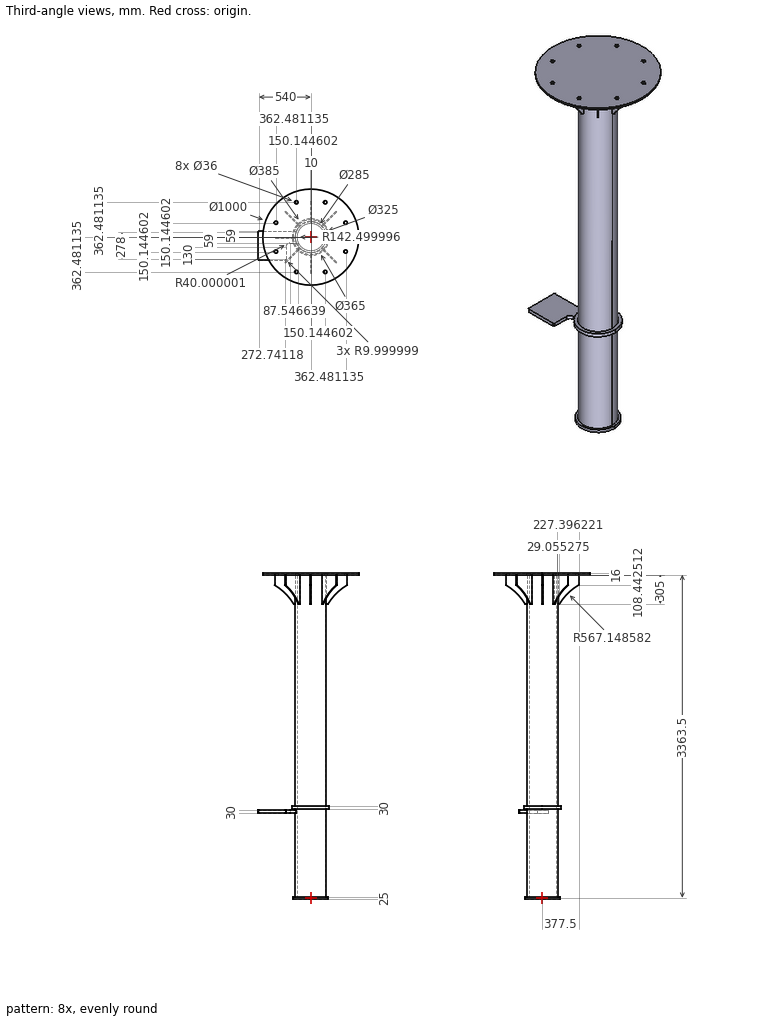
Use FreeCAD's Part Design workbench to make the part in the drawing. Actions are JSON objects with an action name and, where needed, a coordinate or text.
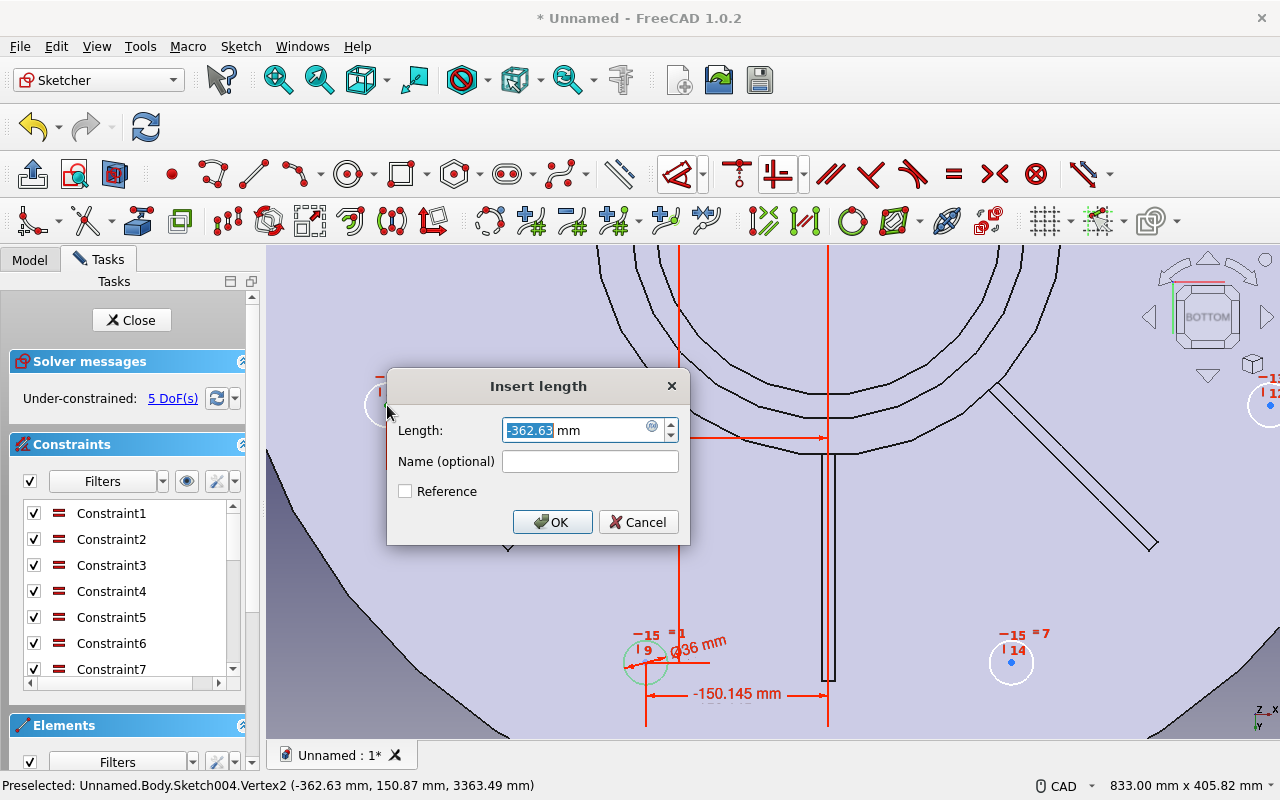
{"action": "type", "text": "-362.481135"}
{"action": "key", "text": "Return"}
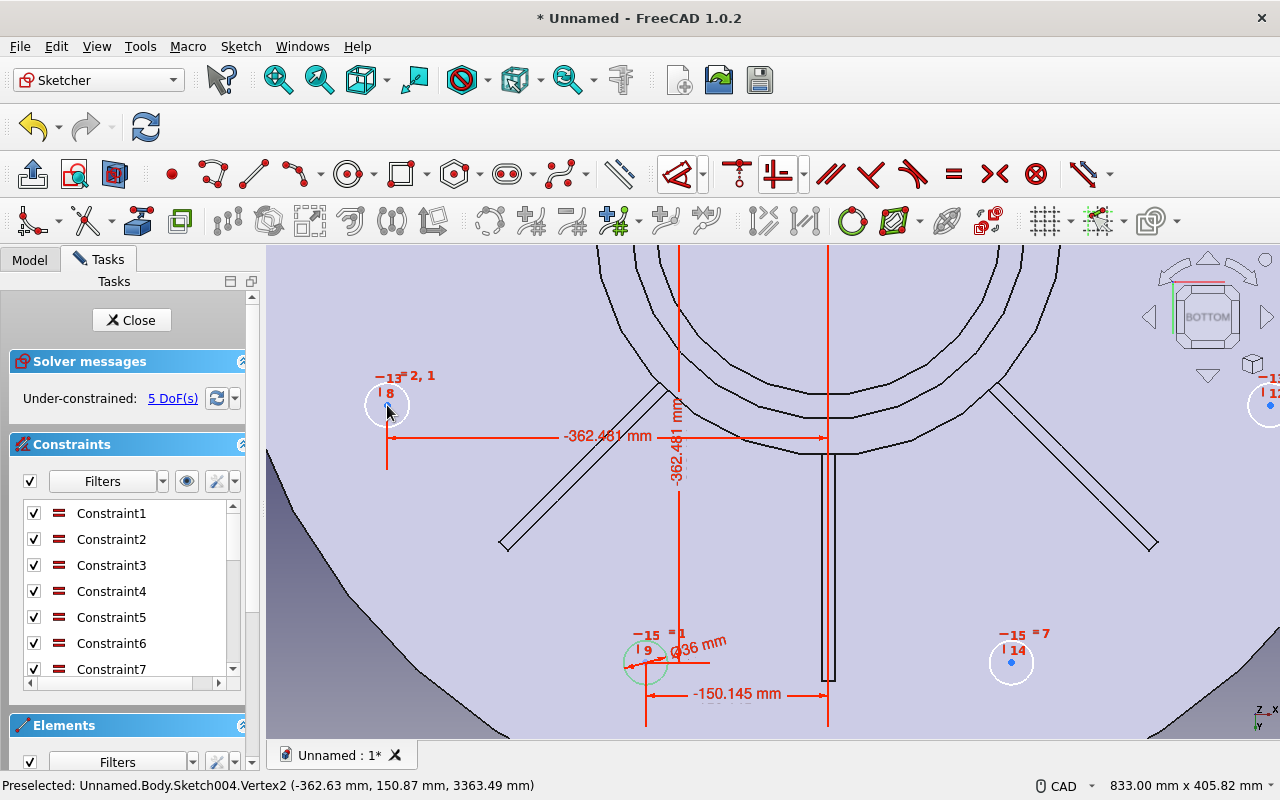
{"action": "left_click", "coordinate": [387, 405]}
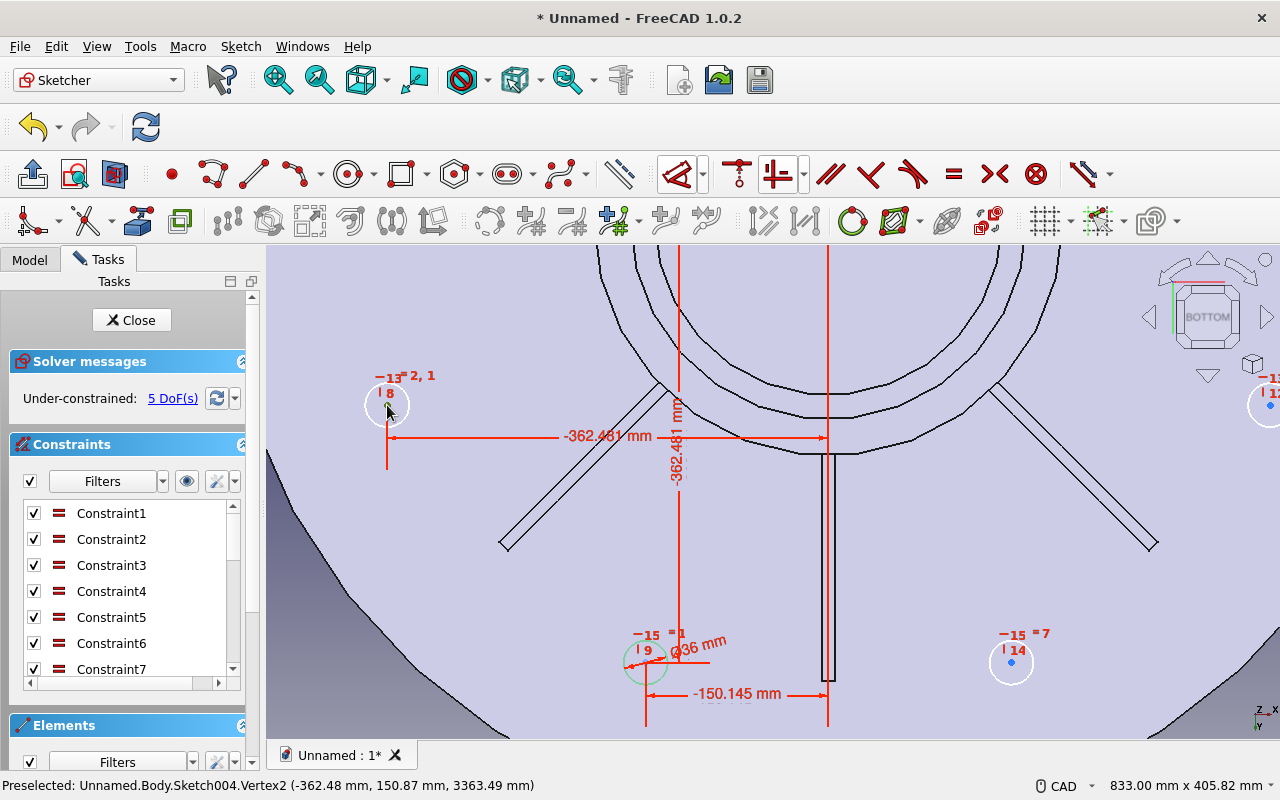
{"action": "key", "text": "i"}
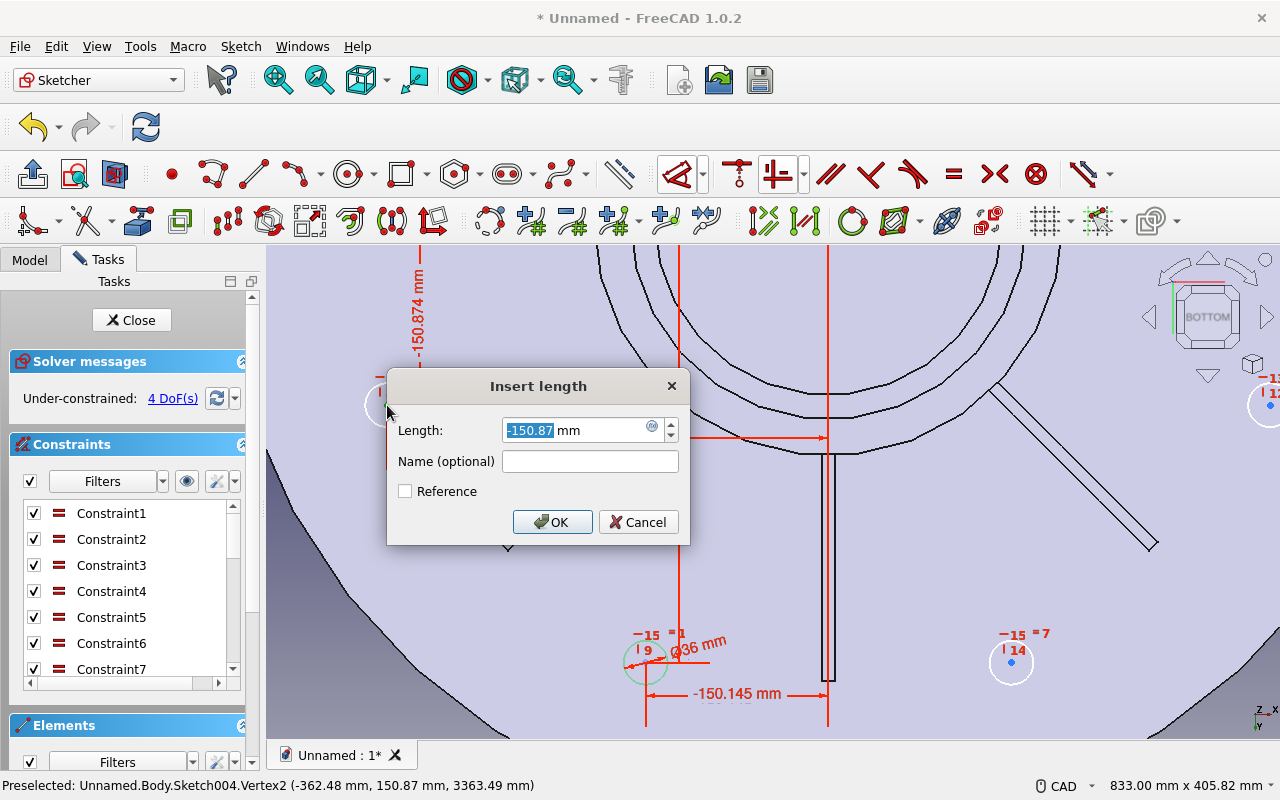
{"action": "type", "text": "-150.144602"}
{"action": "key", "text": "Return"}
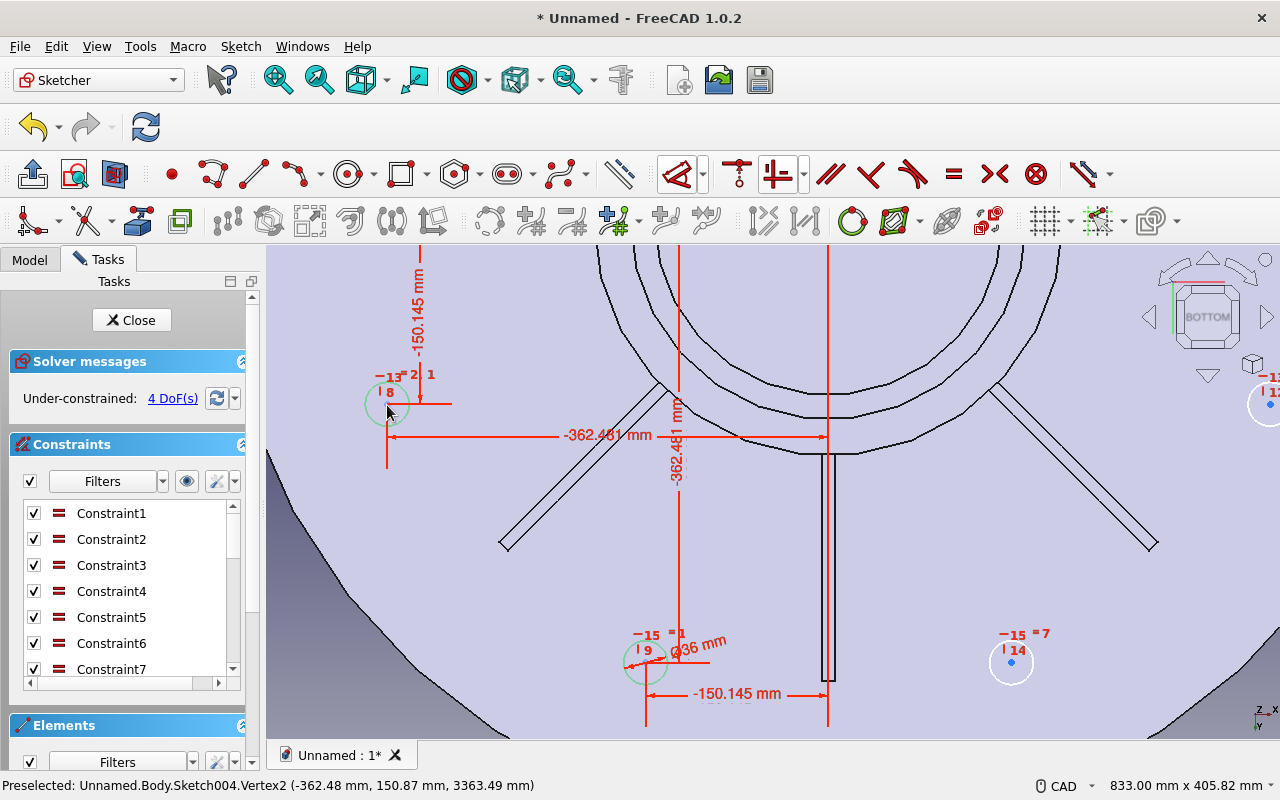
{"action": "scroll", "coordinate": [632, 649], "scroll_direction": "down", "scroll_amount": 5}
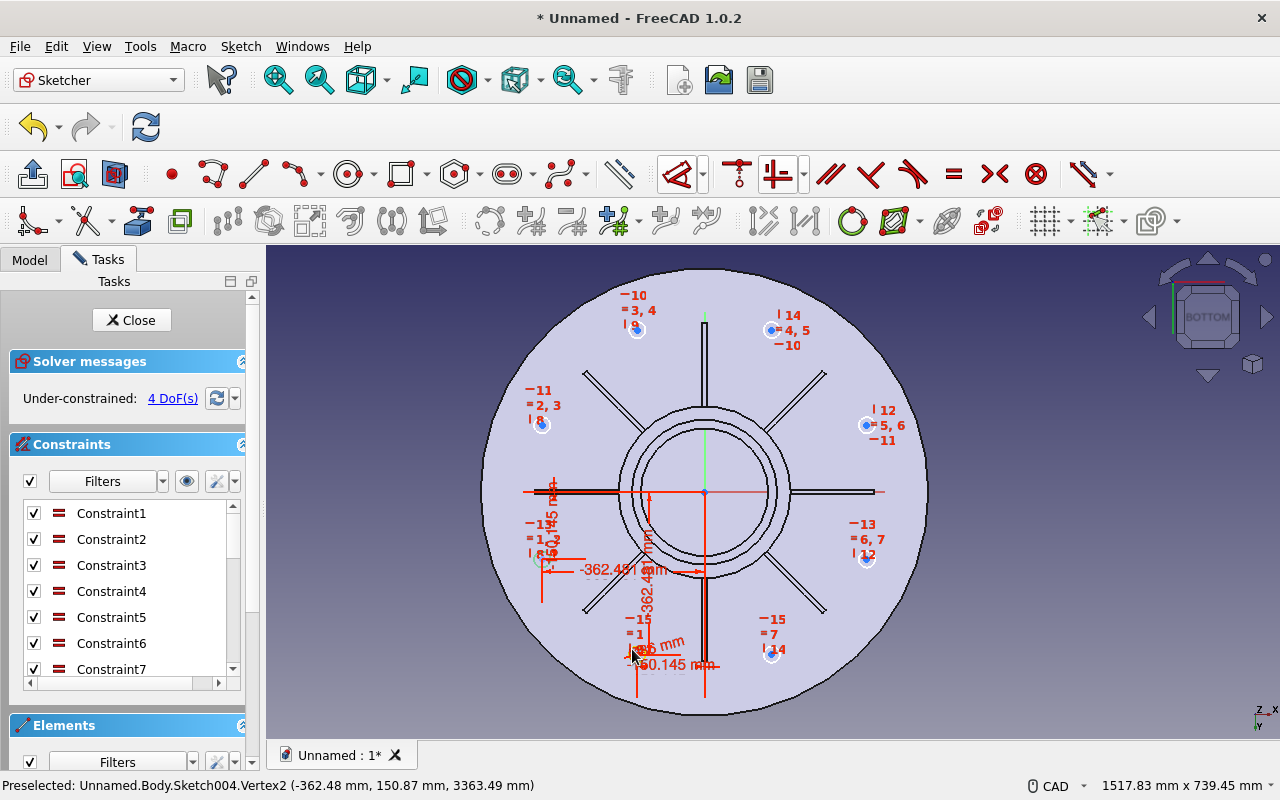
{"action": "left_click", "coordinate": [542, 425]}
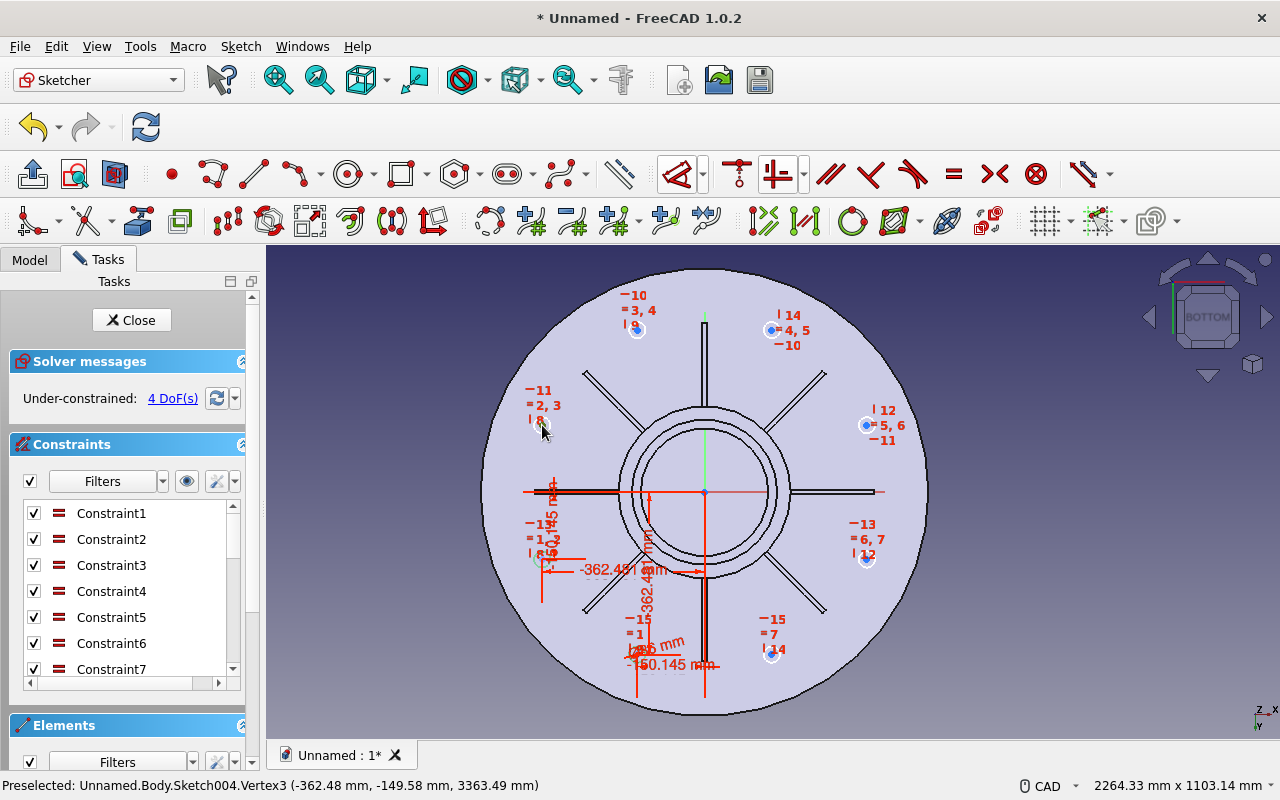
{"action": "key", "text": "i"}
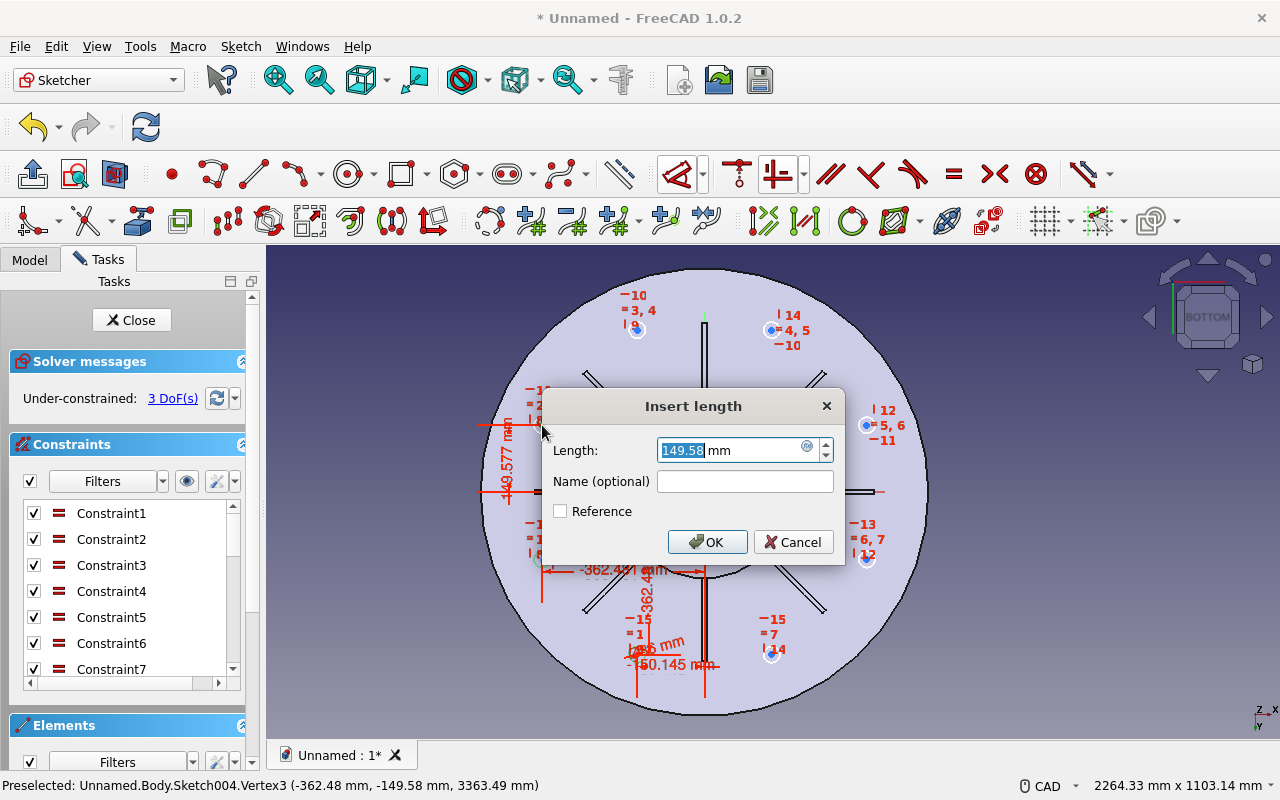
{"action": "type", "text": "150.144602"}
{"action": "key", "text": "Return"}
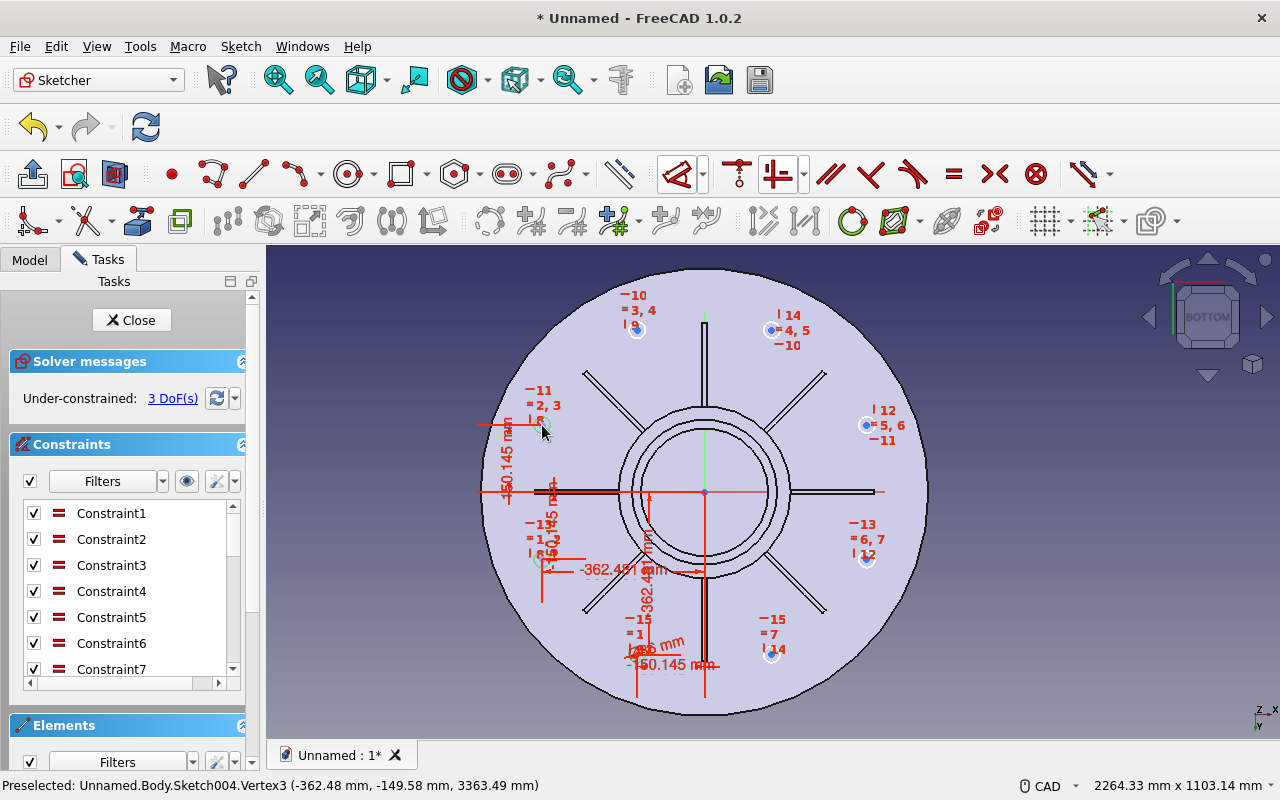
{"action": "left_click", "coordinate": [637, 330]}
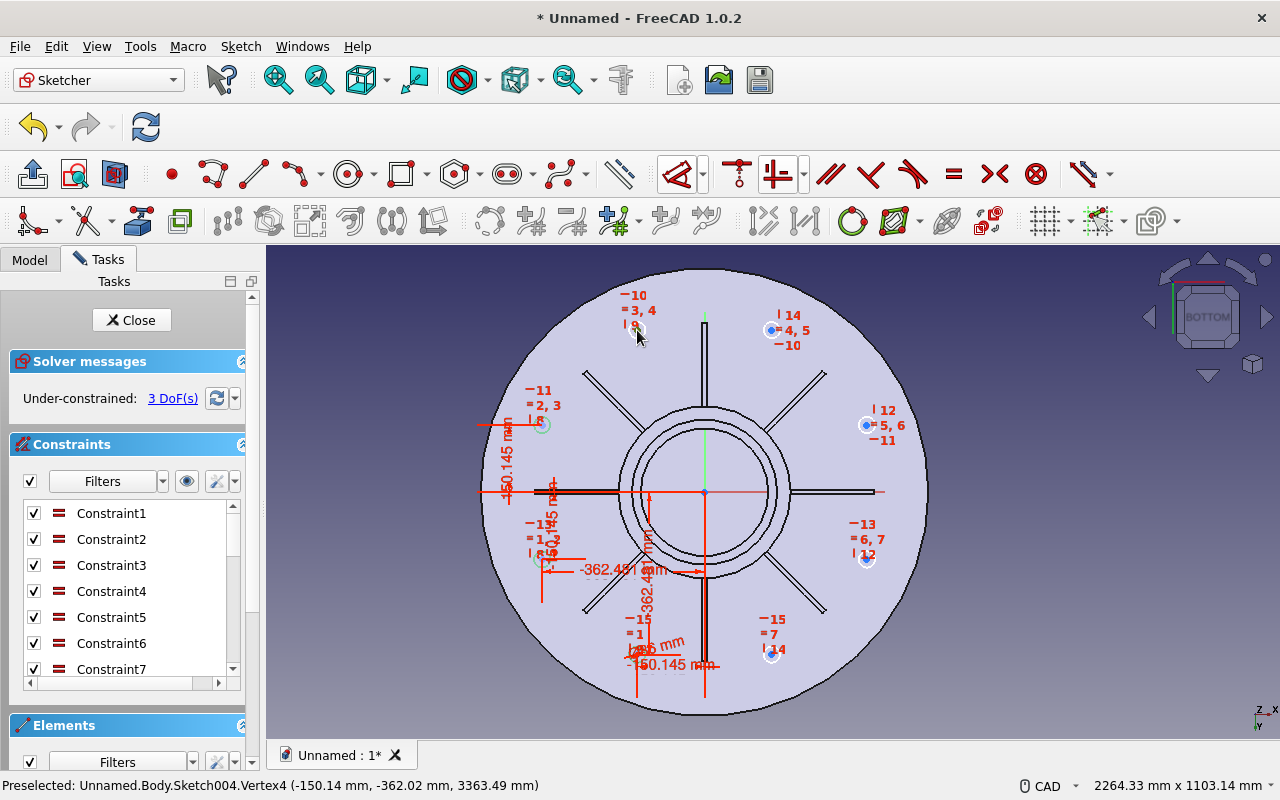
{"action": "key", "text": "i"}